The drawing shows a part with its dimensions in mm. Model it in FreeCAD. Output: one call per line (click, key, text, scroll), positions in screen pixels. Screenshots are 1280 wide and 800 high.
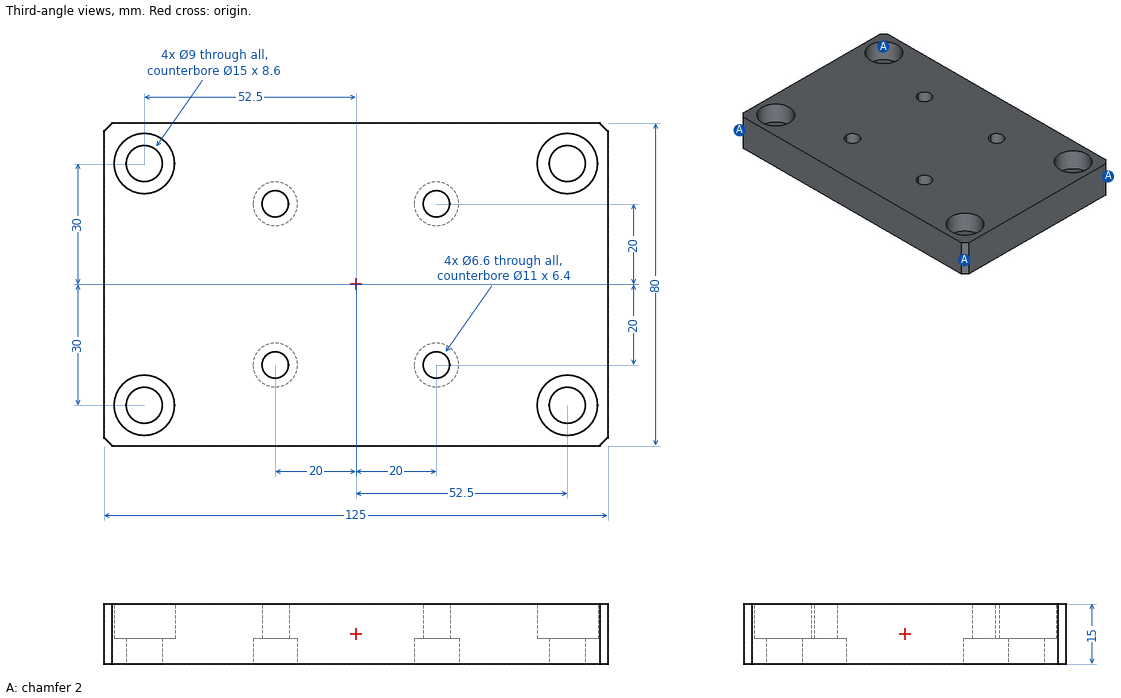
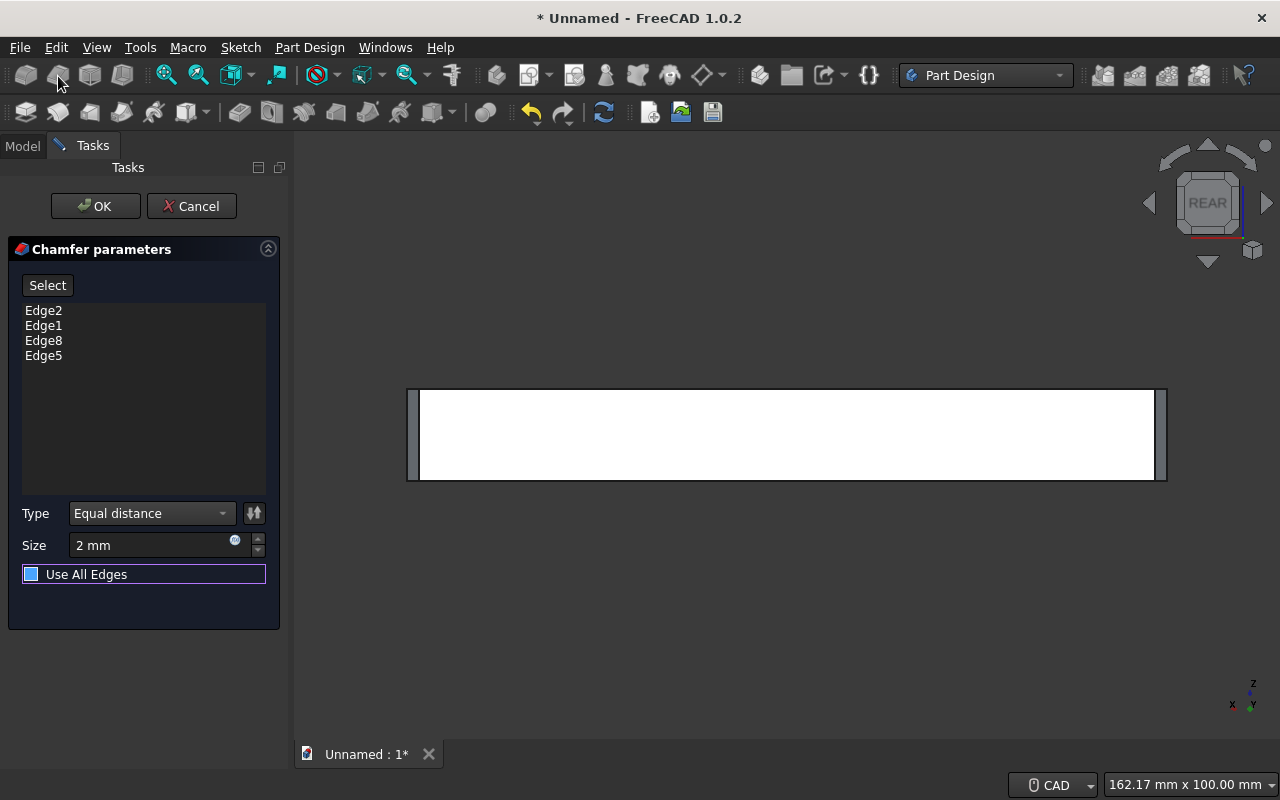
click(96, 206)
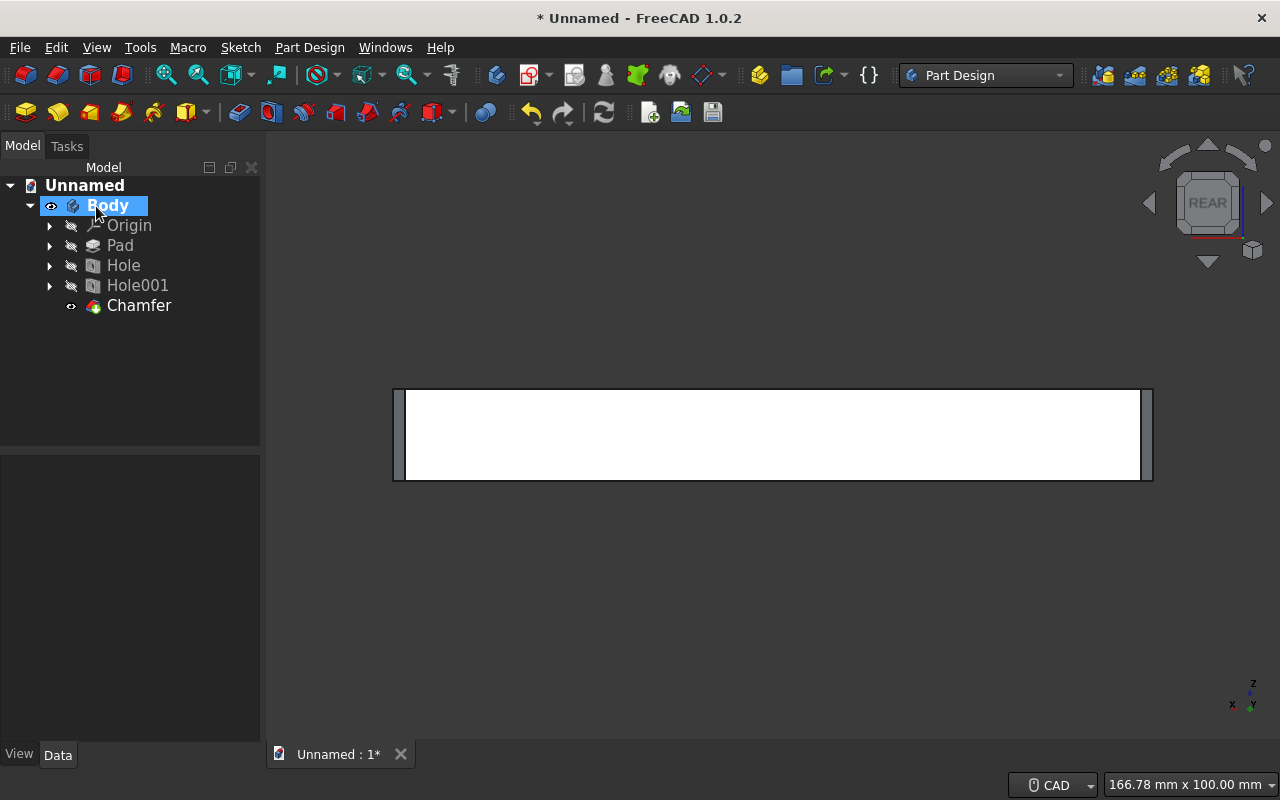
key(0)